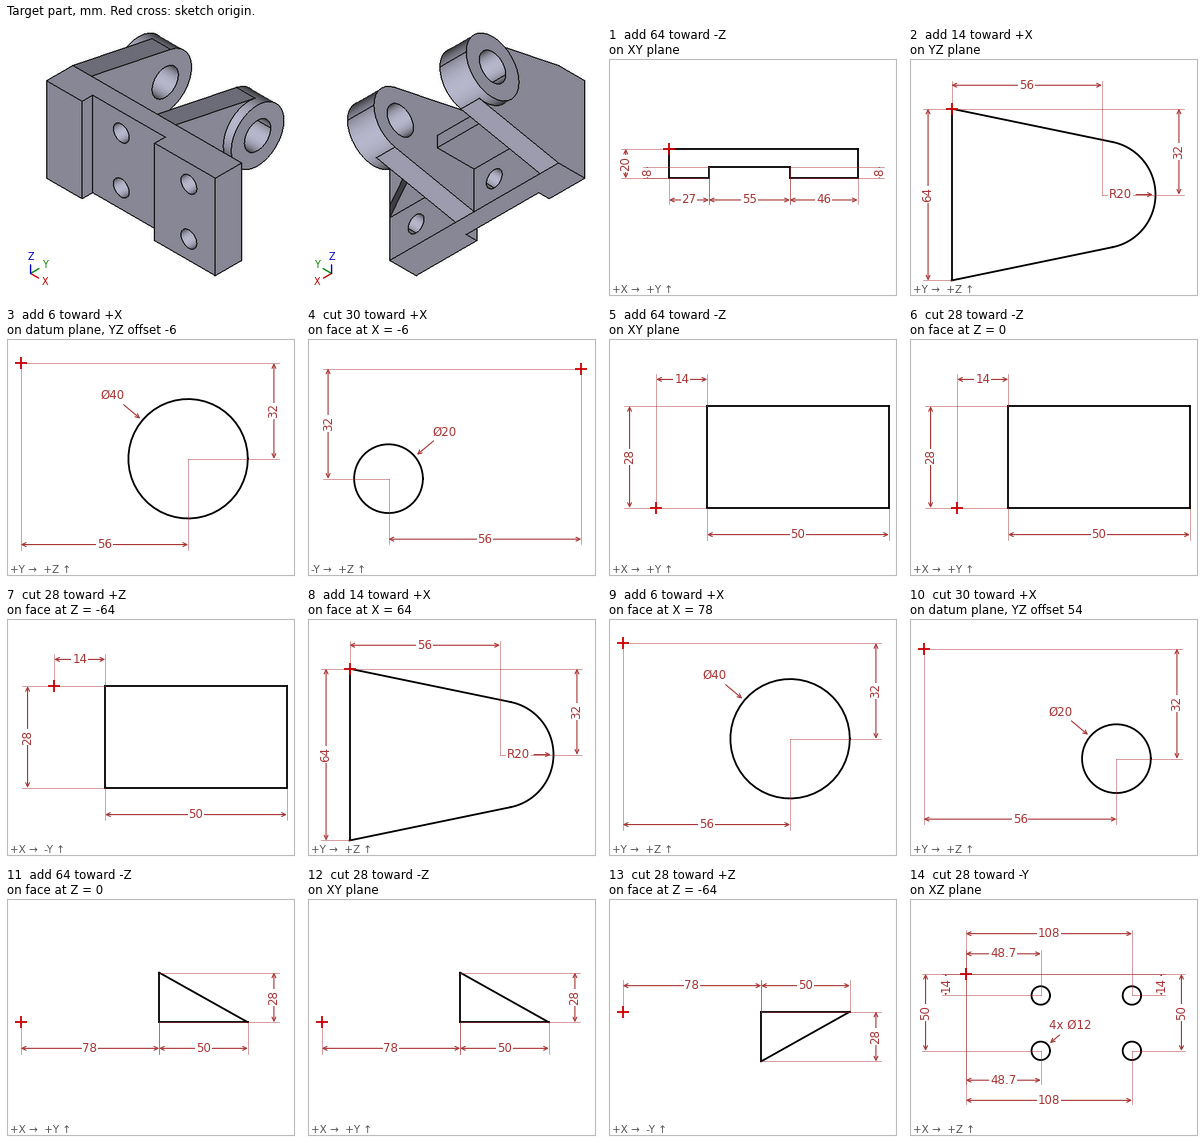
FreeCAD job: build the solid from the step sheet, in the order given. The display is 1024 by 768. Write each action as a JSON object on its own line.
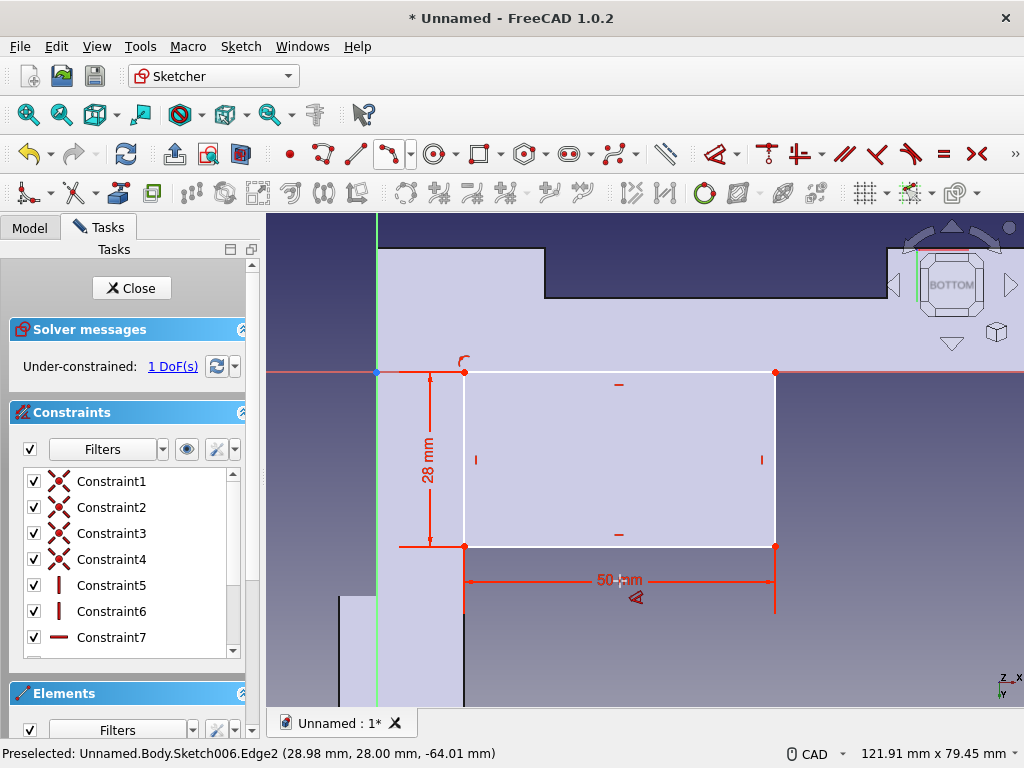
{"action": "left_click", "coordinate": [464, 372]}
{"action": "left_click", "coordinate": [420, 338]}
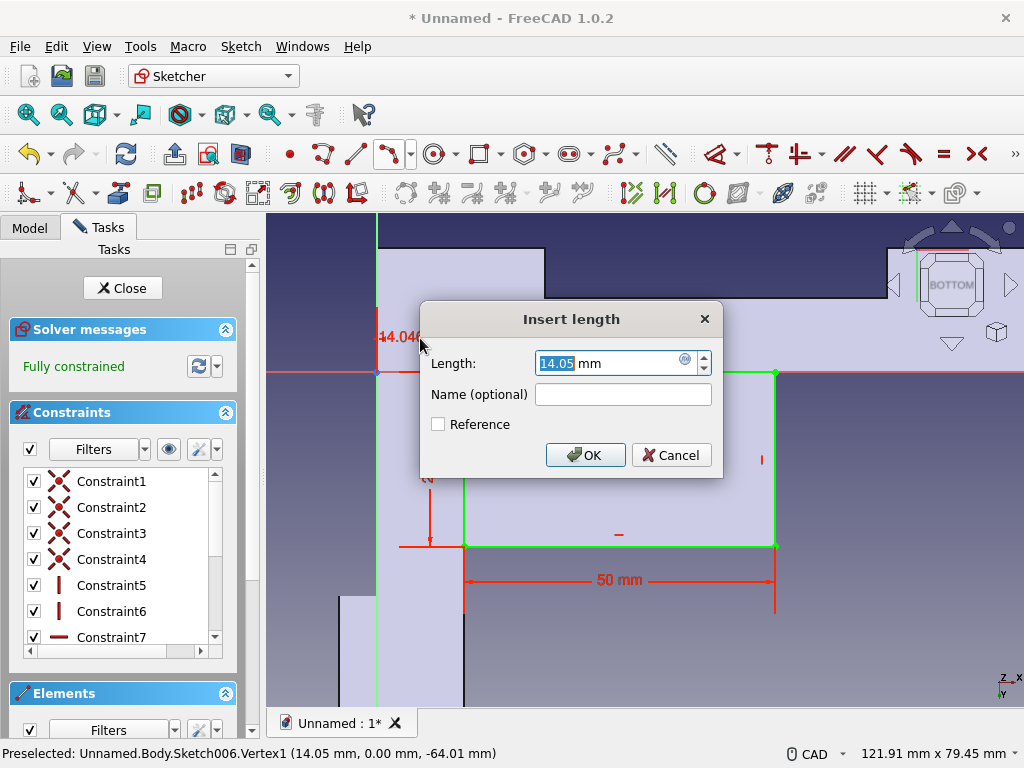
{"action": "type", "text": "14"}
{"action": "key", "text": "Return"}
{"action": "key", "text": "Escape"}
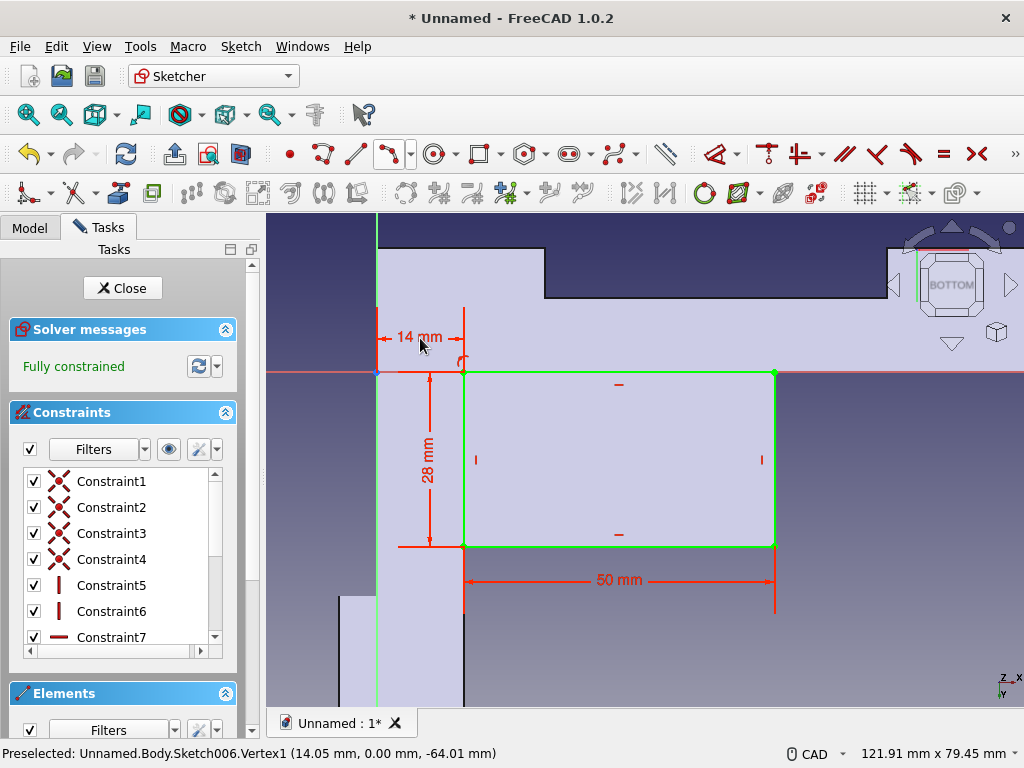
{"action": "left_click", "coordinate": [123, 288]}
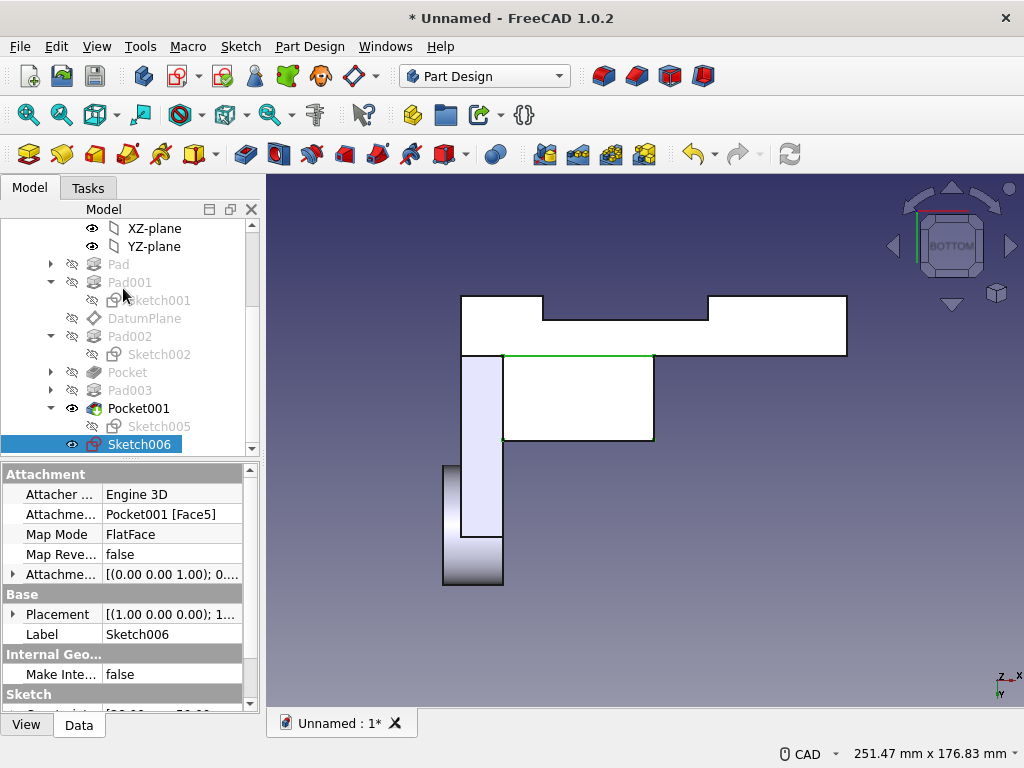
{"action": "left_click", "coordinate": [246, 154]}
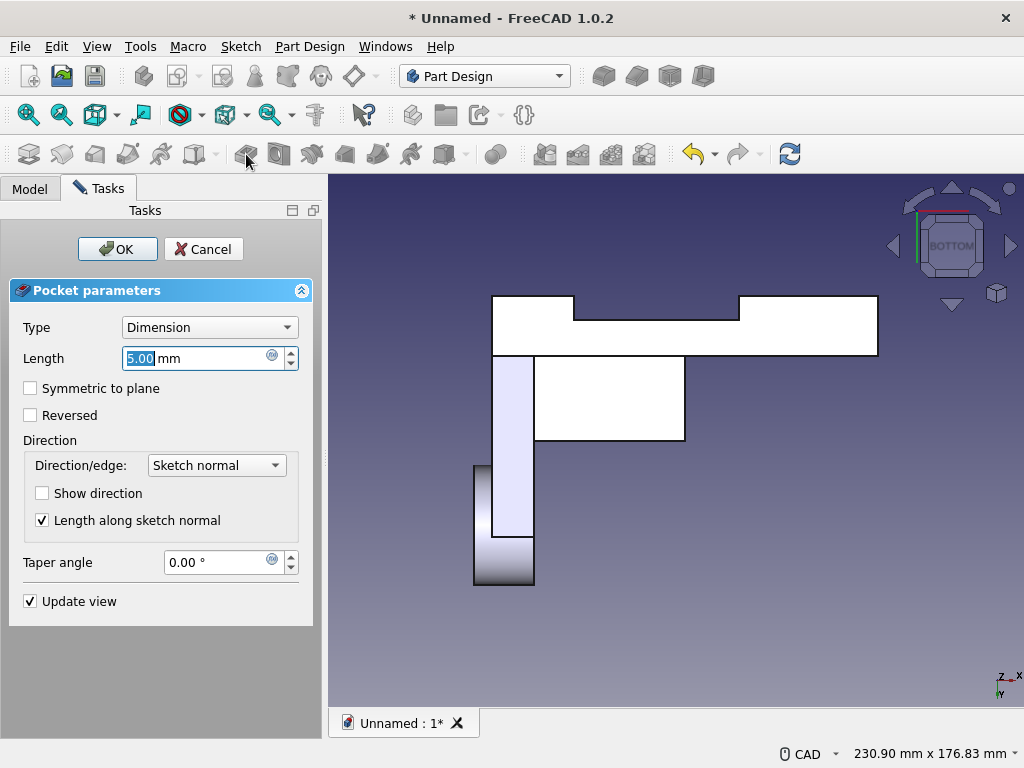
{"action": "type", "text": "28"}
{"action": "key", "text": "Tab"}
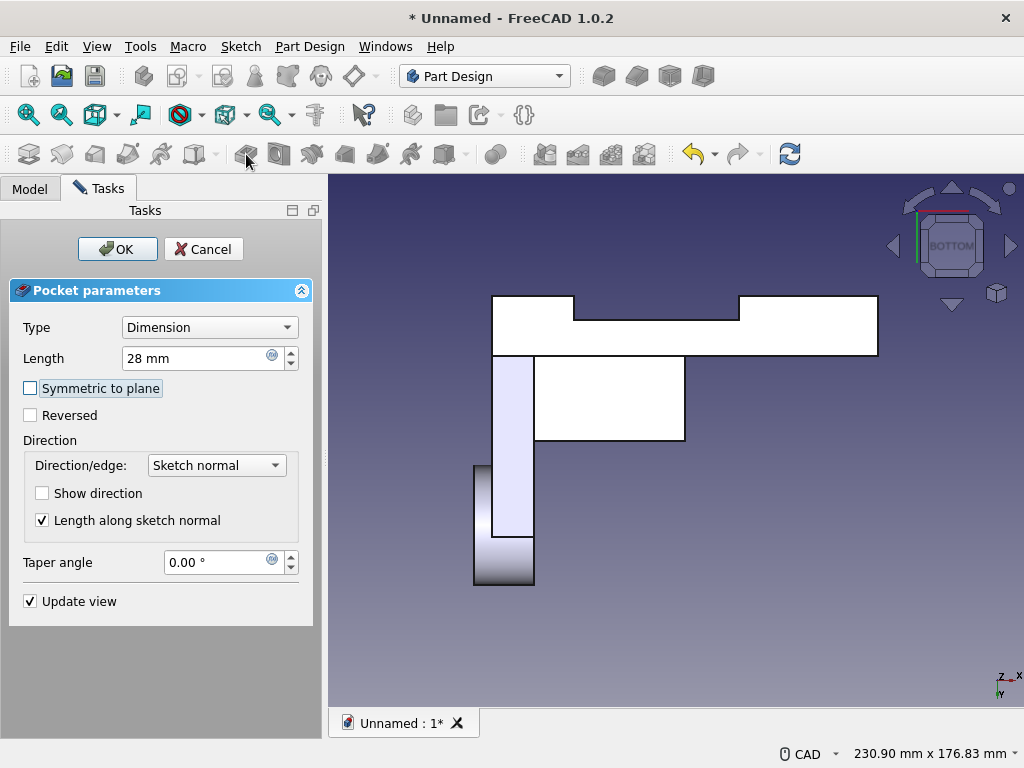
{"action": "left_click", "coordinate": [118, 249]}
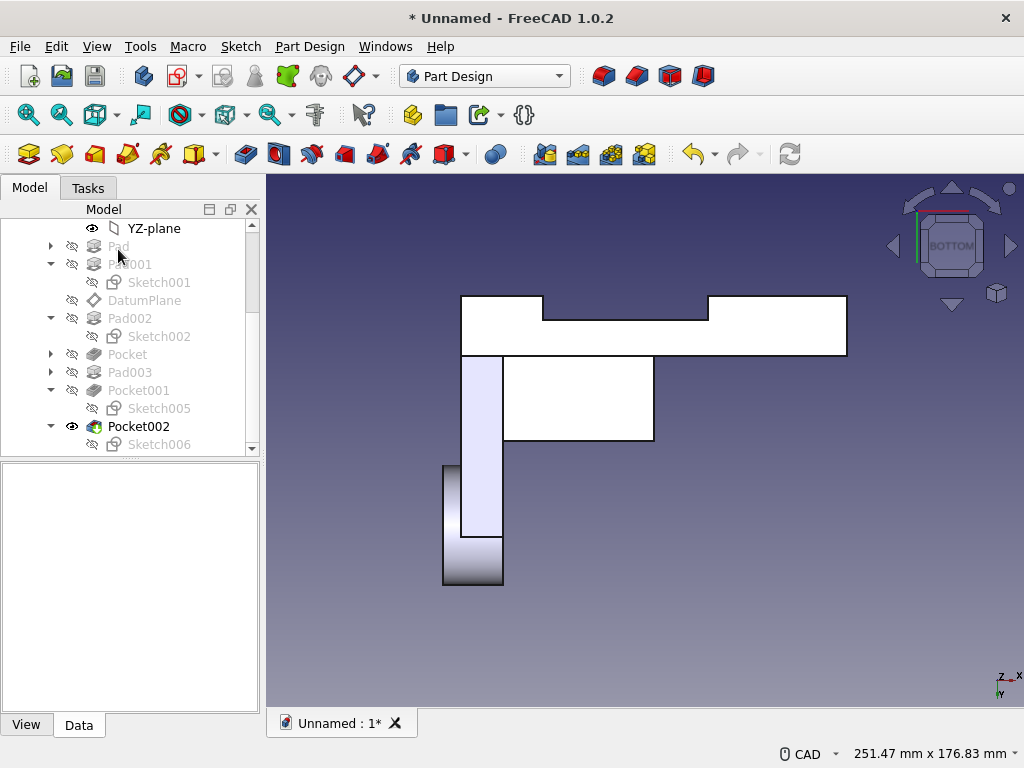
{"action": "key", "text": "0"}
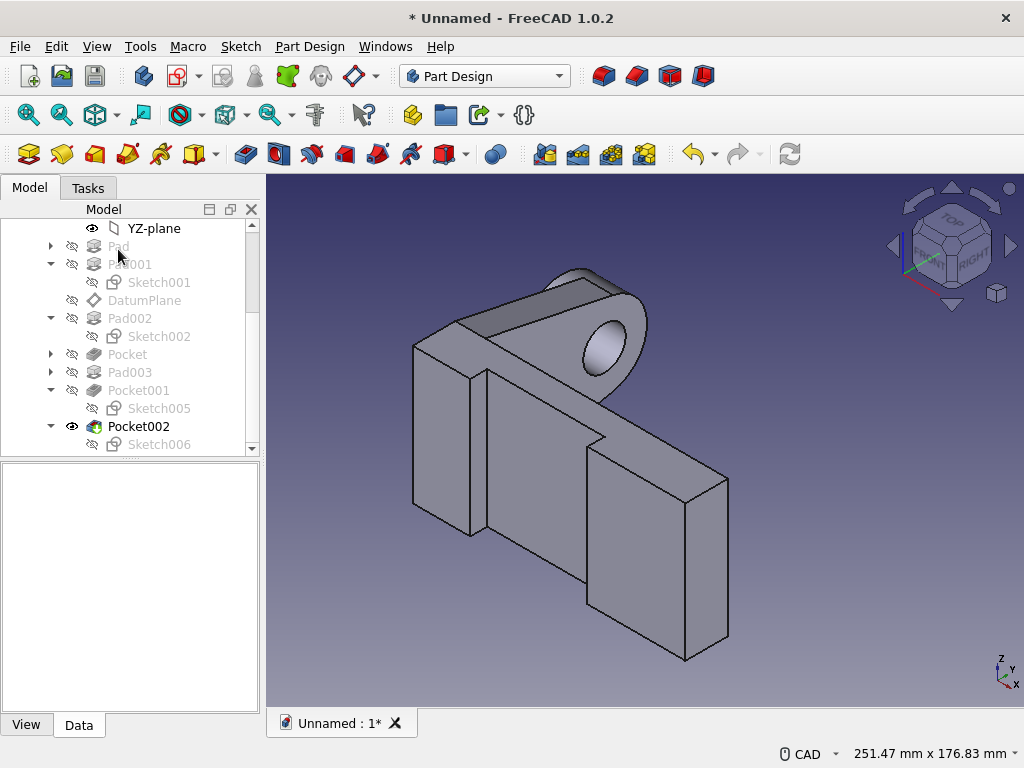
{"action": "key", "text": "3"}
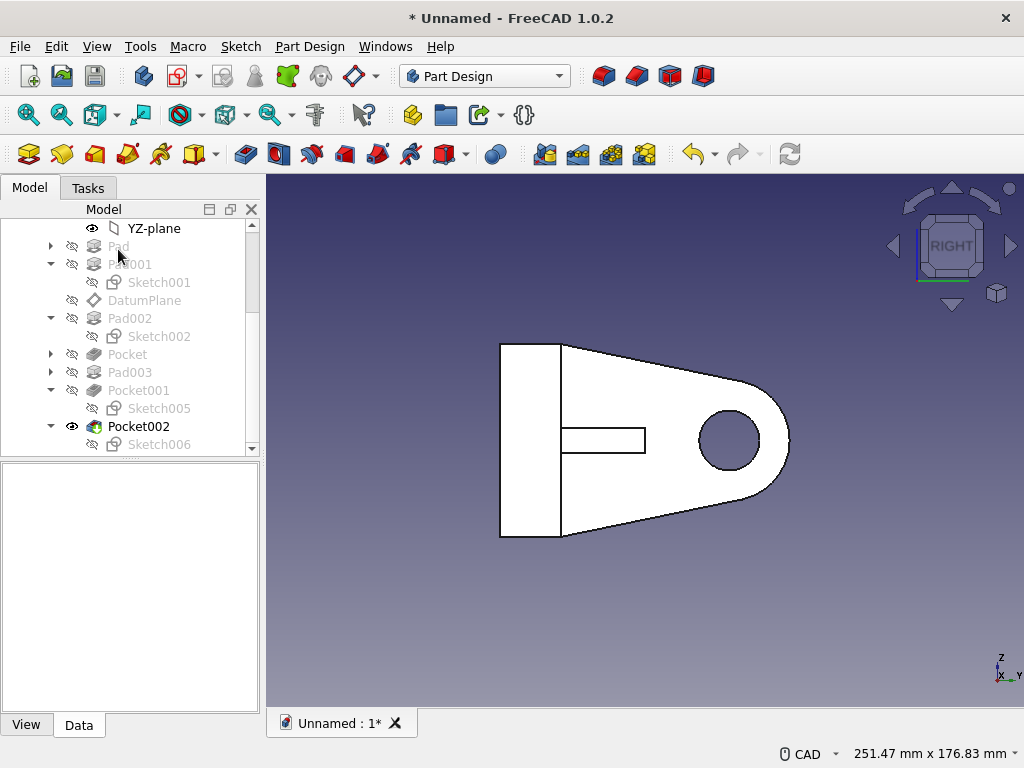
{"action": "left_click", "coordinate": [29, 116]}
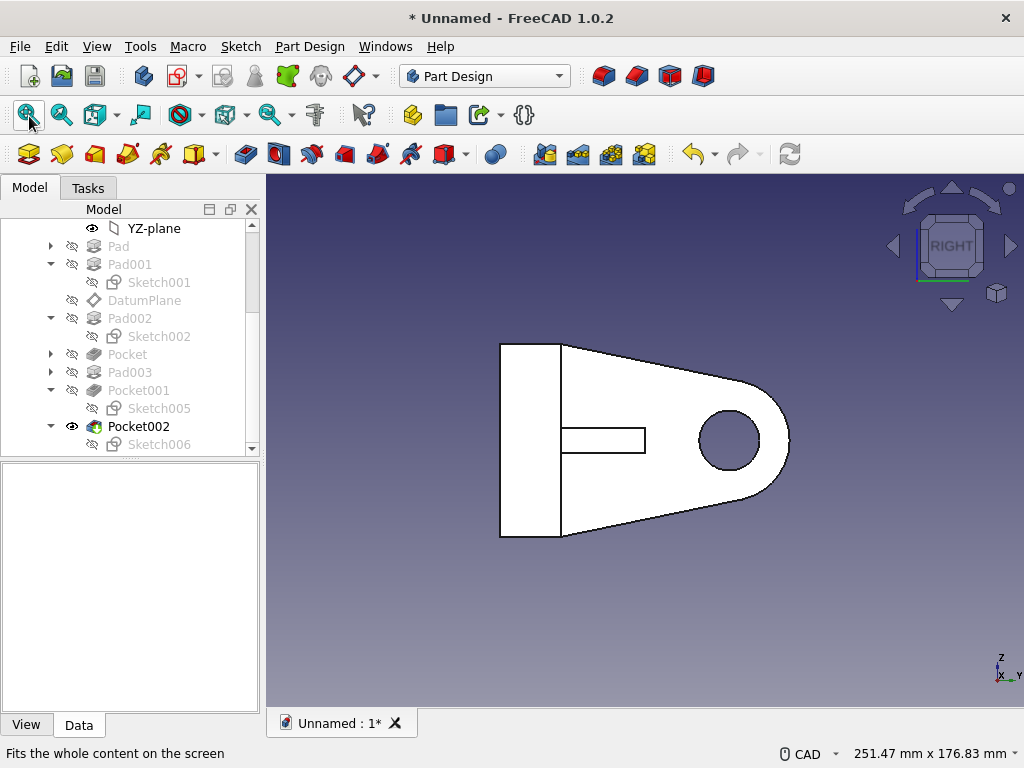
{"action": "left_click", "coordinate": [627, 439]}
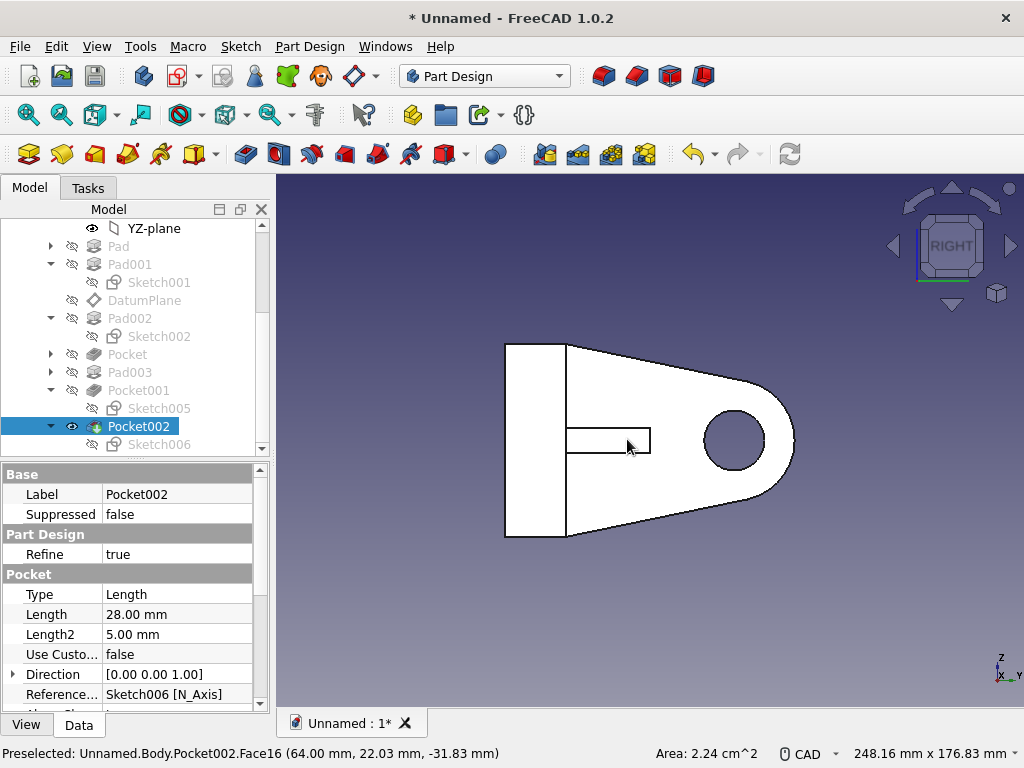
{"action": "left_click", "coordinate": [176, 76]}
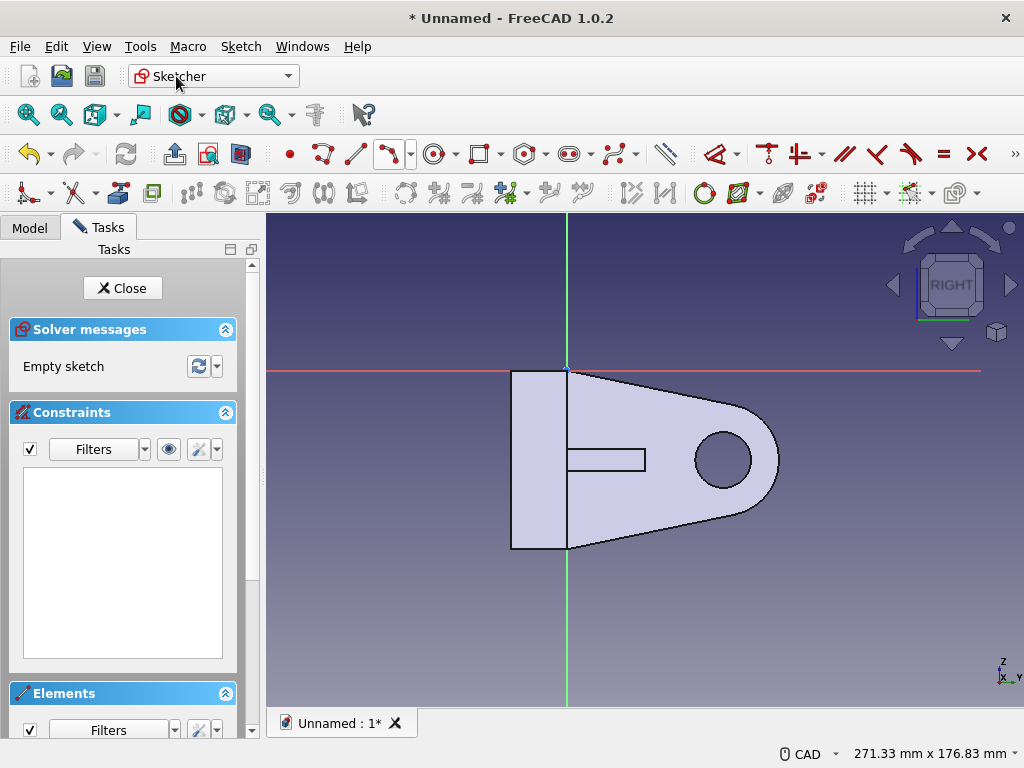
{"action": "scroll", "coordinate": [790, 460], "scroll_direction": "up", "scroll_amount": 3}